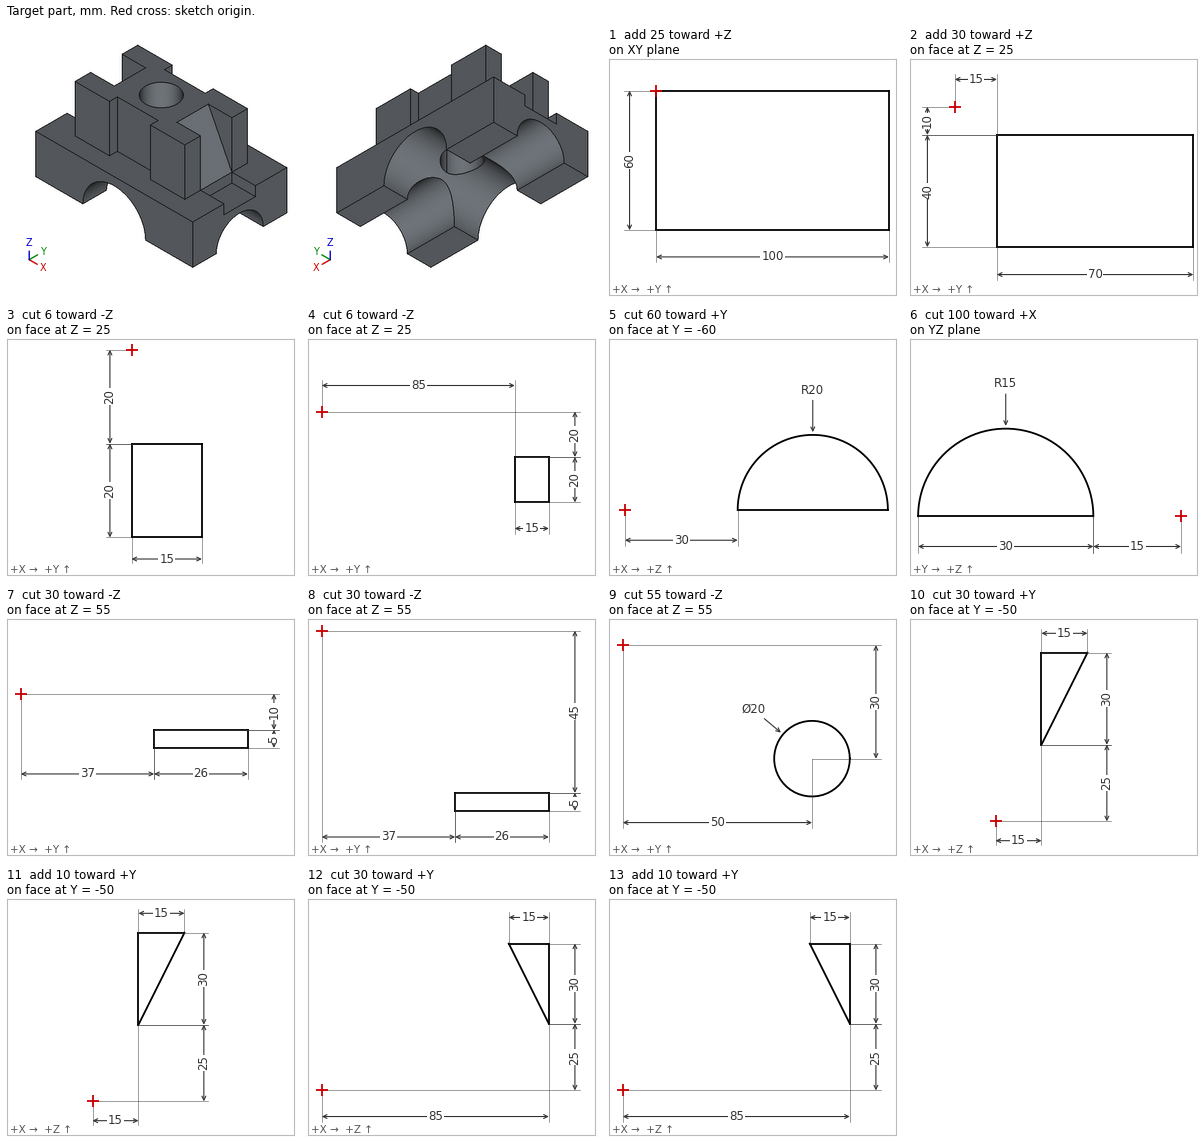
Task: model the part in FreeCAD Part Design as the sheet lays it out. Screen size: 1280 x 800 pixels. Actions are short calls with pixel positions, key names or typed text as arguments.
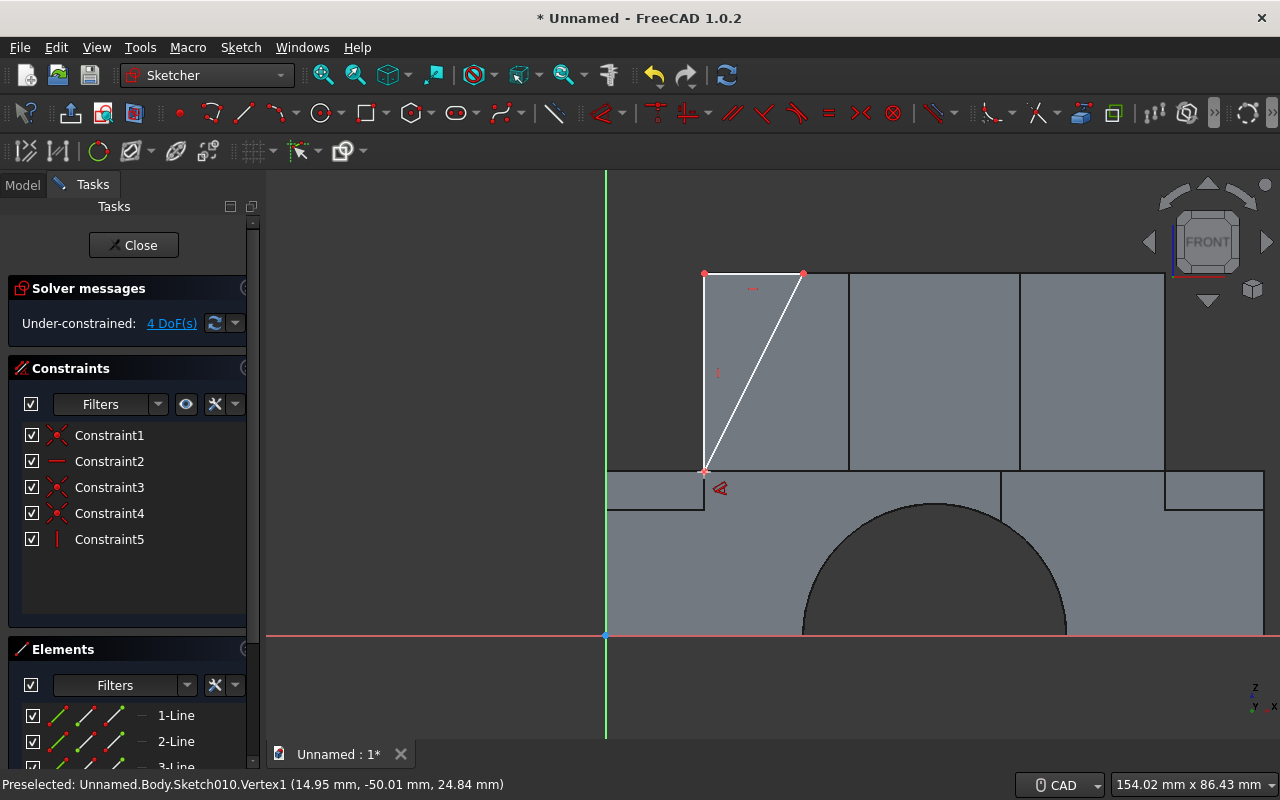
click(773, 274)
click(753, 240)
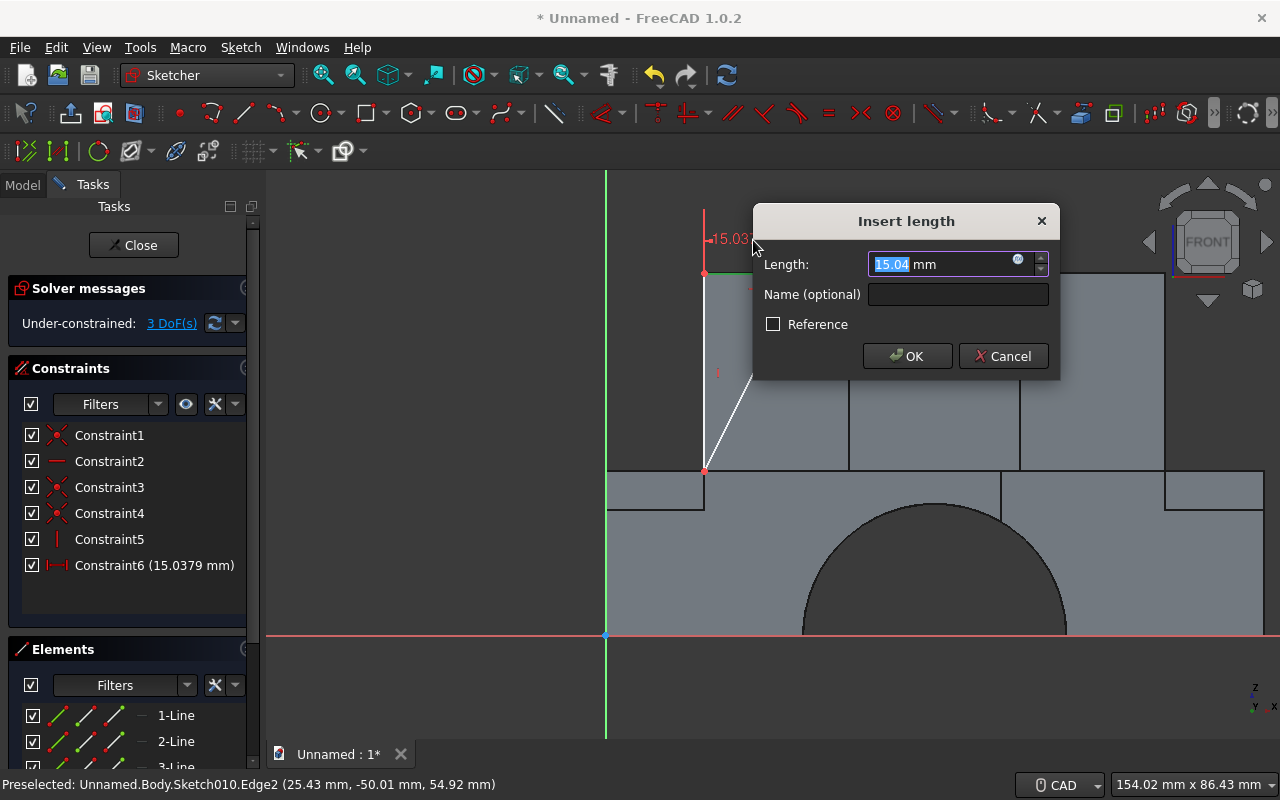
text(15)
key(Return)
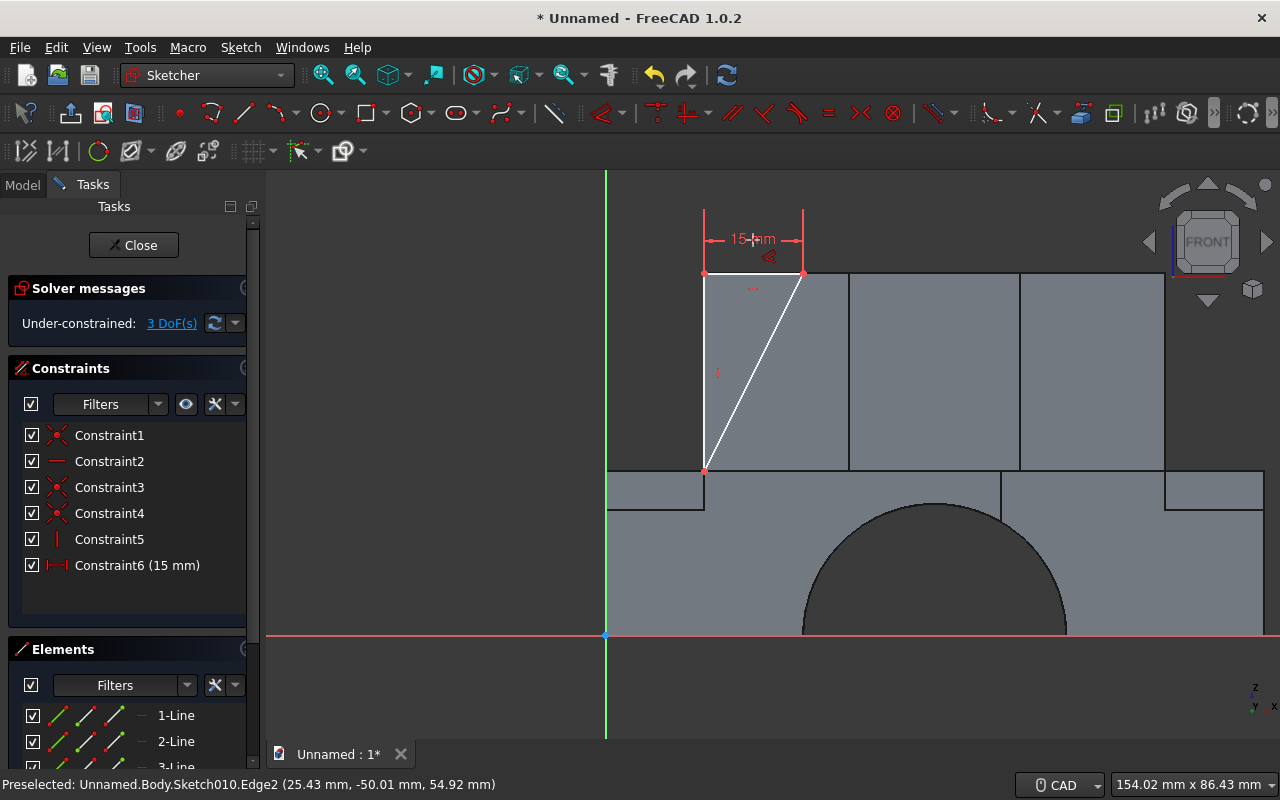
click(704, 333)
click(670, 373)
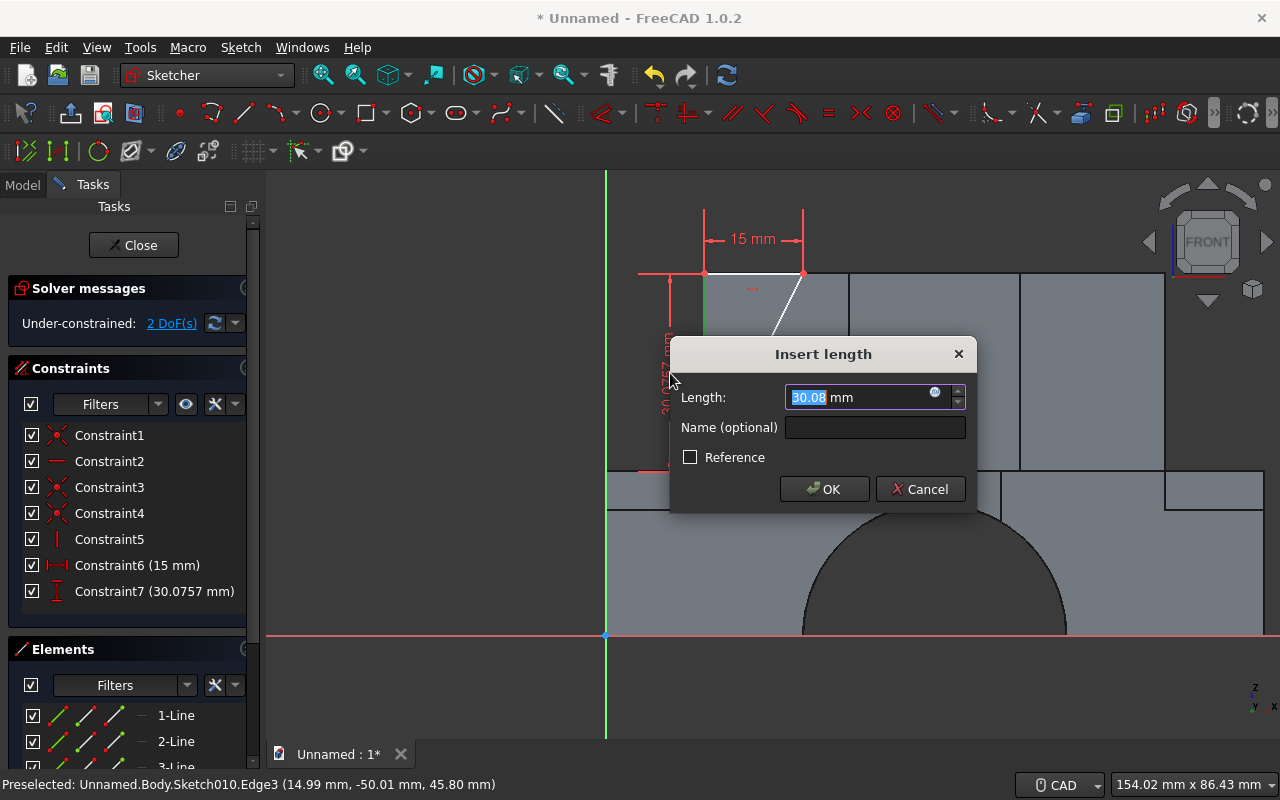
text(30)
key(Return)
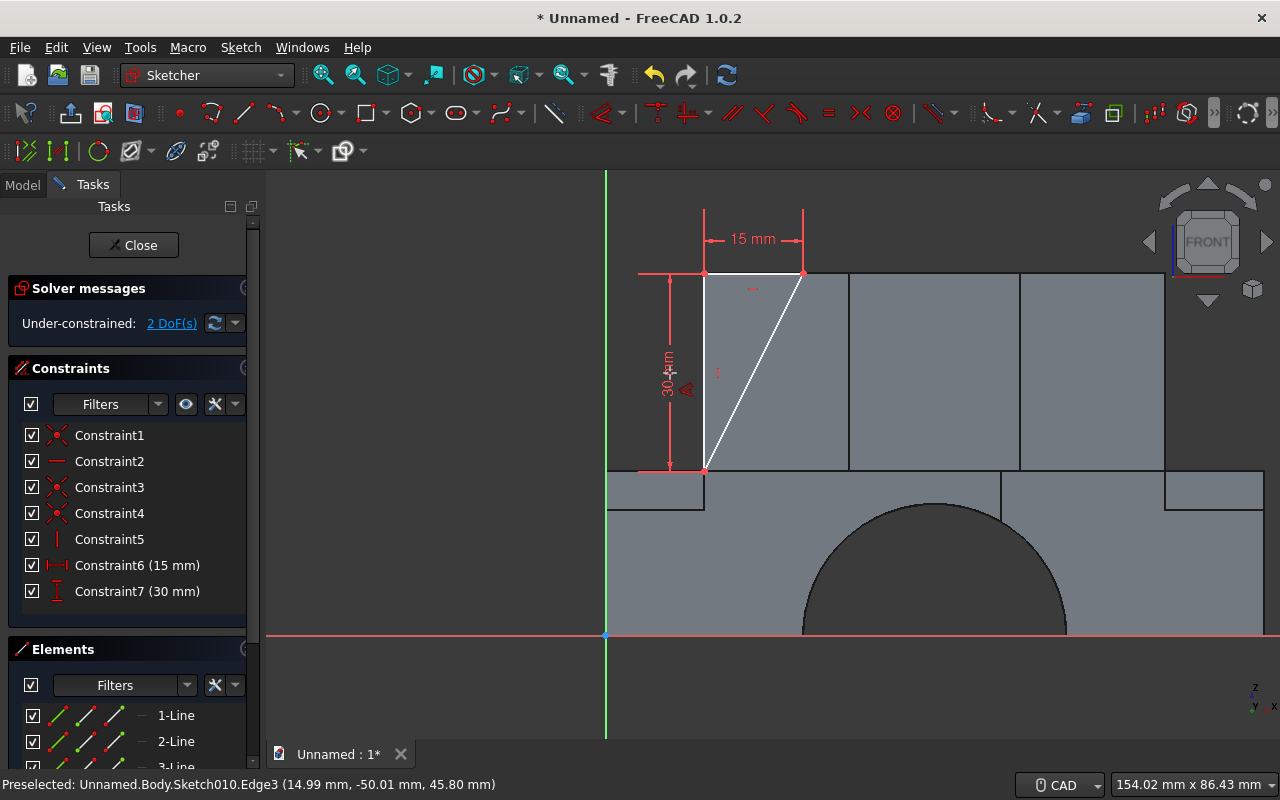
click(704, 472)
click(655, 670)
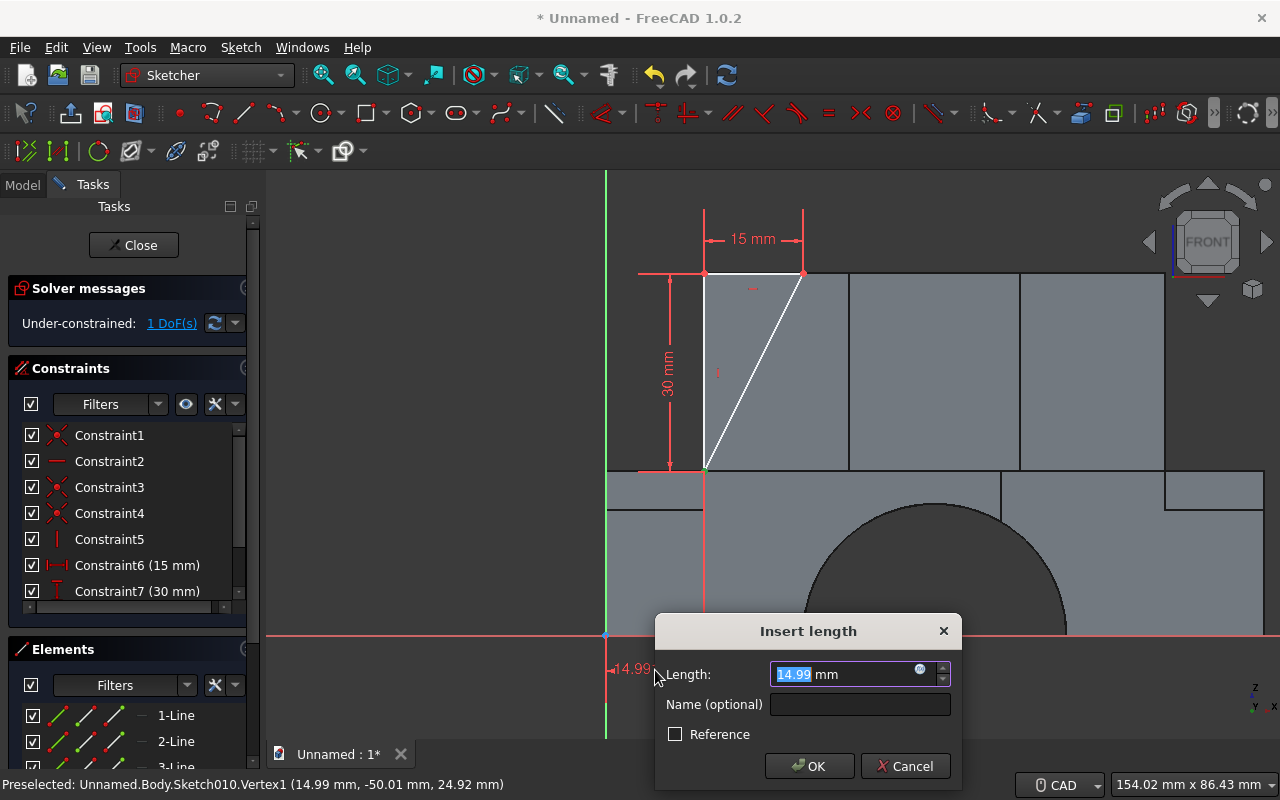
text(15)
key(Return)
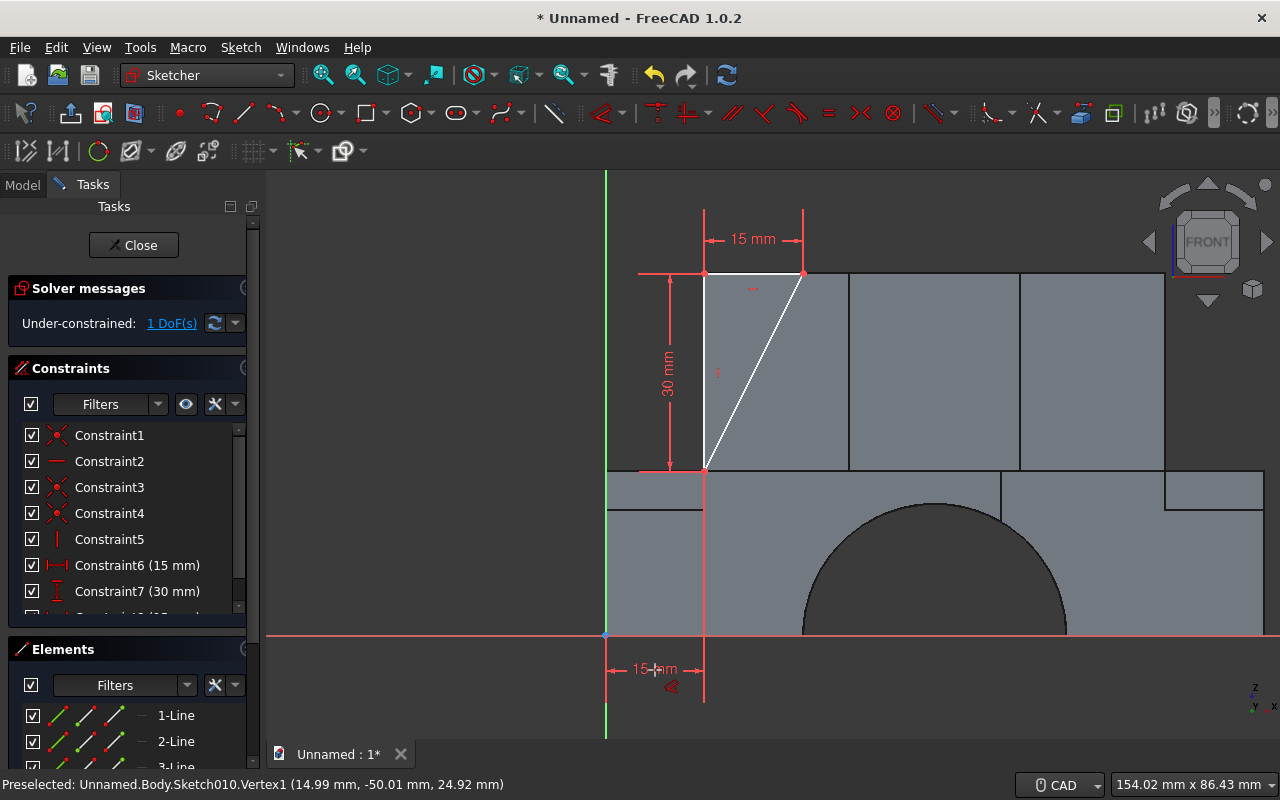
click(704, 472)
click(572, 554)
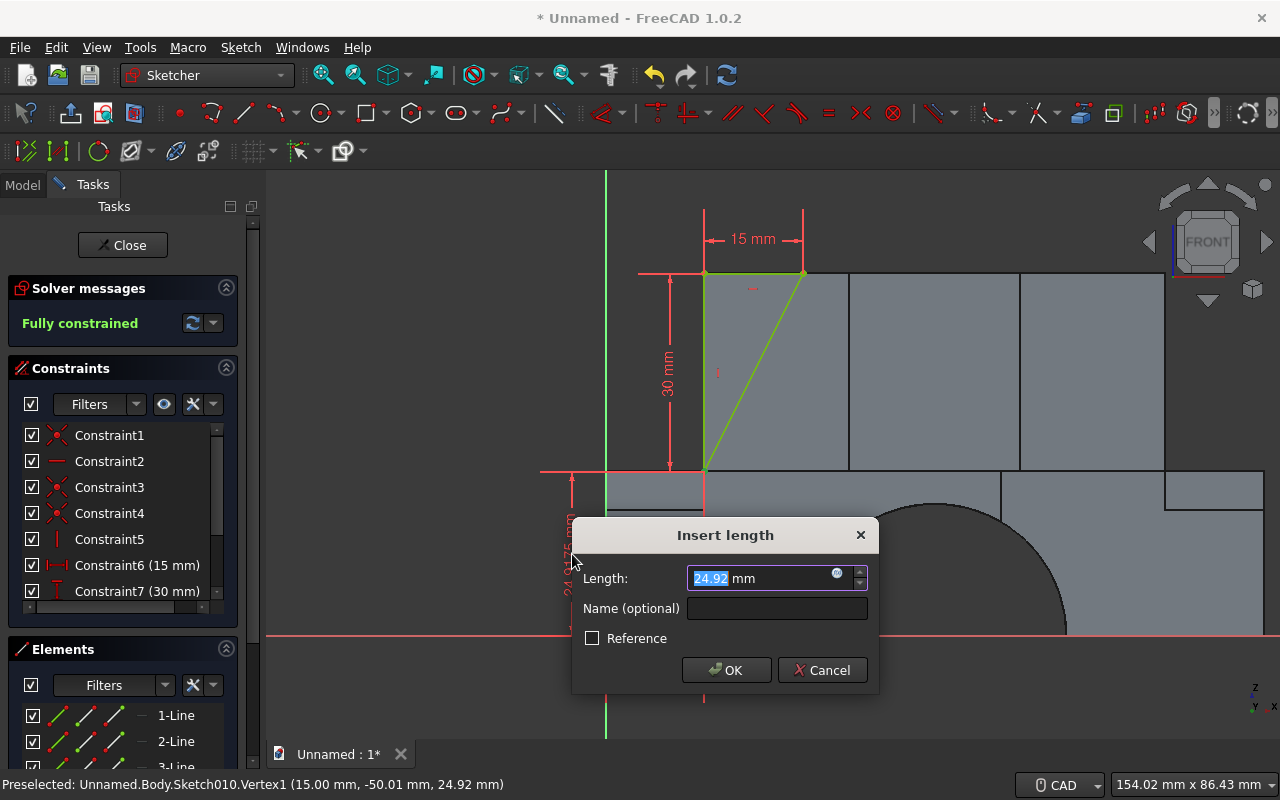
text(25)
key(Return)
key(Escape)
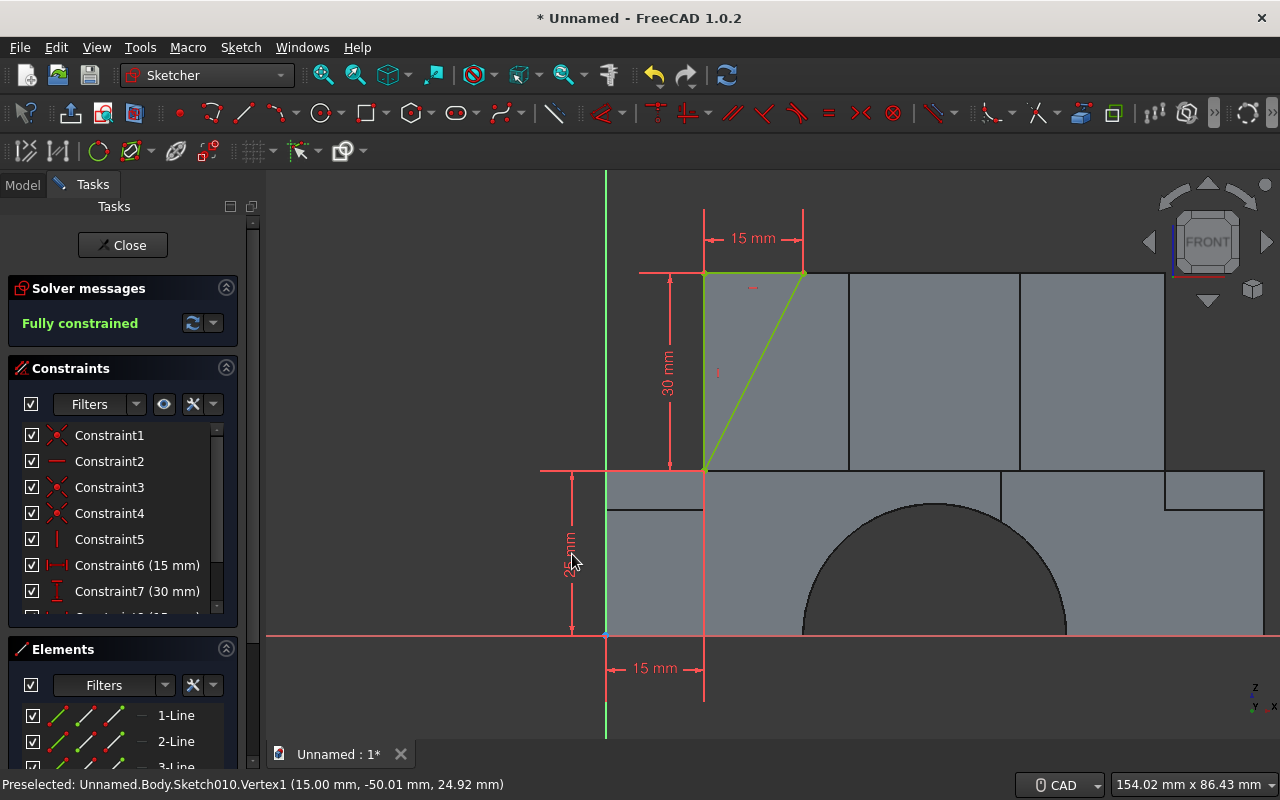
click(123, 245)